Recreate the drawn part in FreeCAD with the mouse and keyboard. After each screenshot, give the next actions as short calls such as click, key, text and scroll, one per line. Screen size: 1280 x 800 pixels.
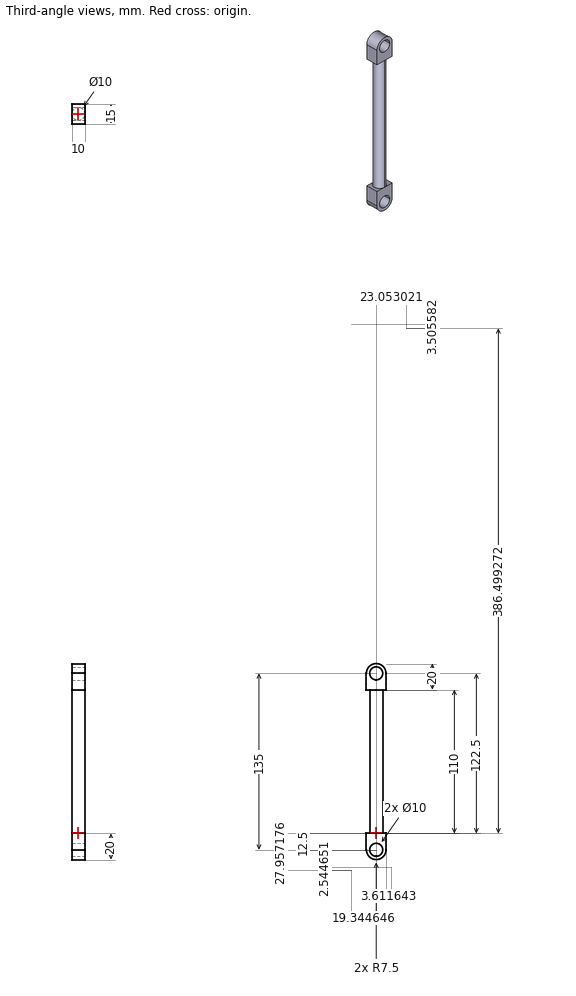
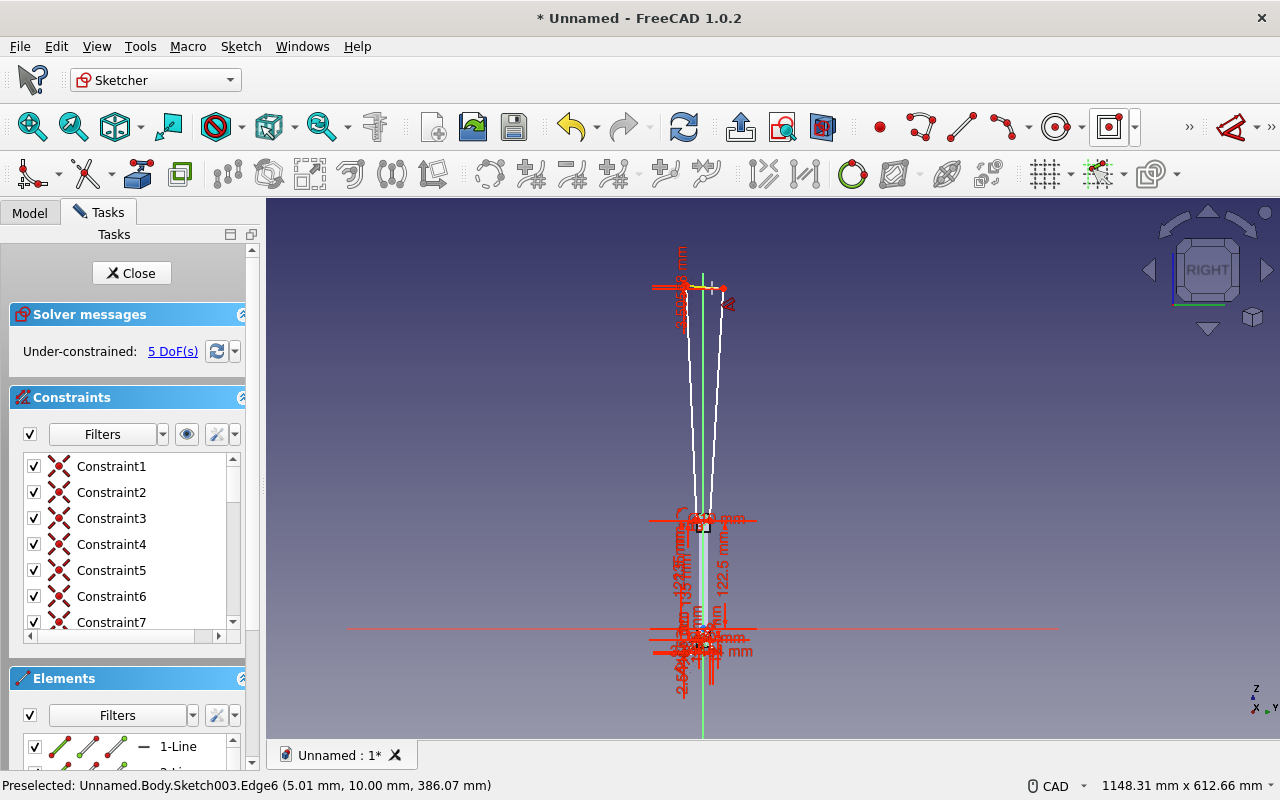
scroll(686, 654, up, 5)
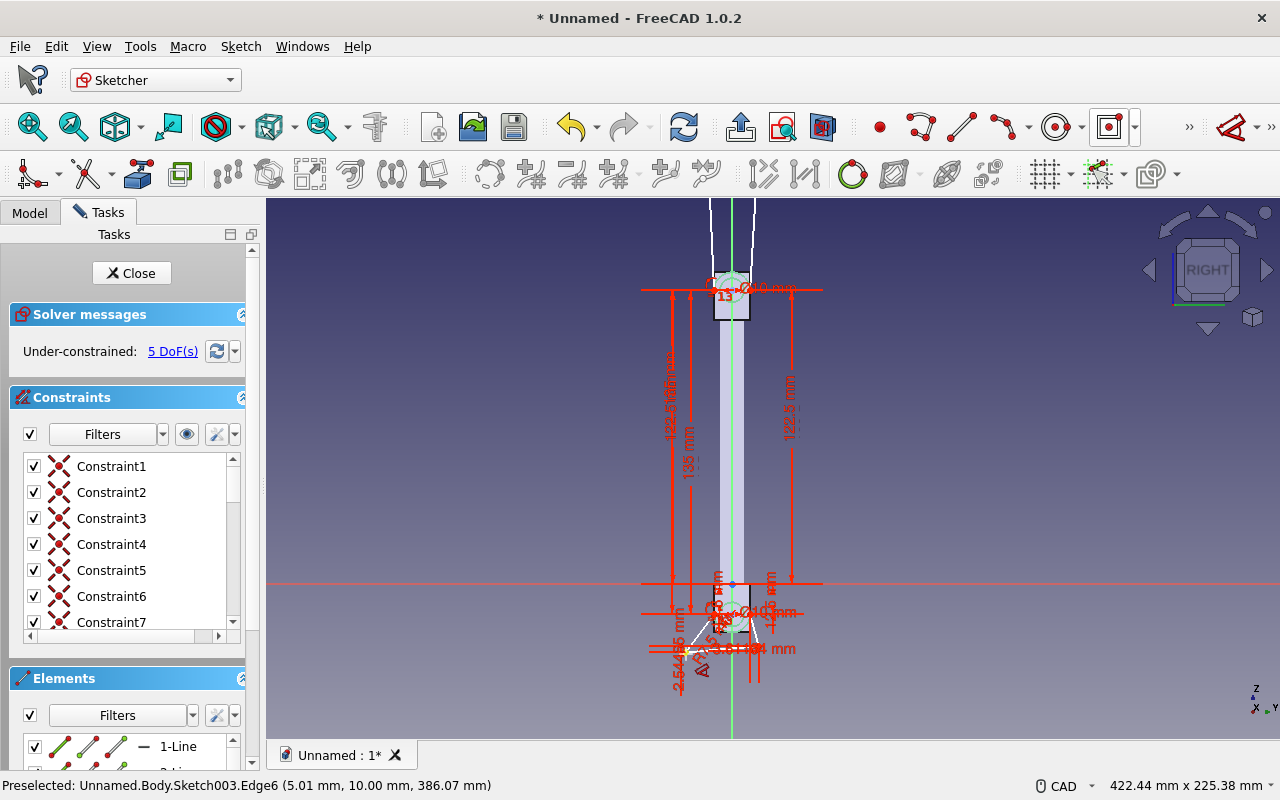
click(686, 652)
click(709, 686)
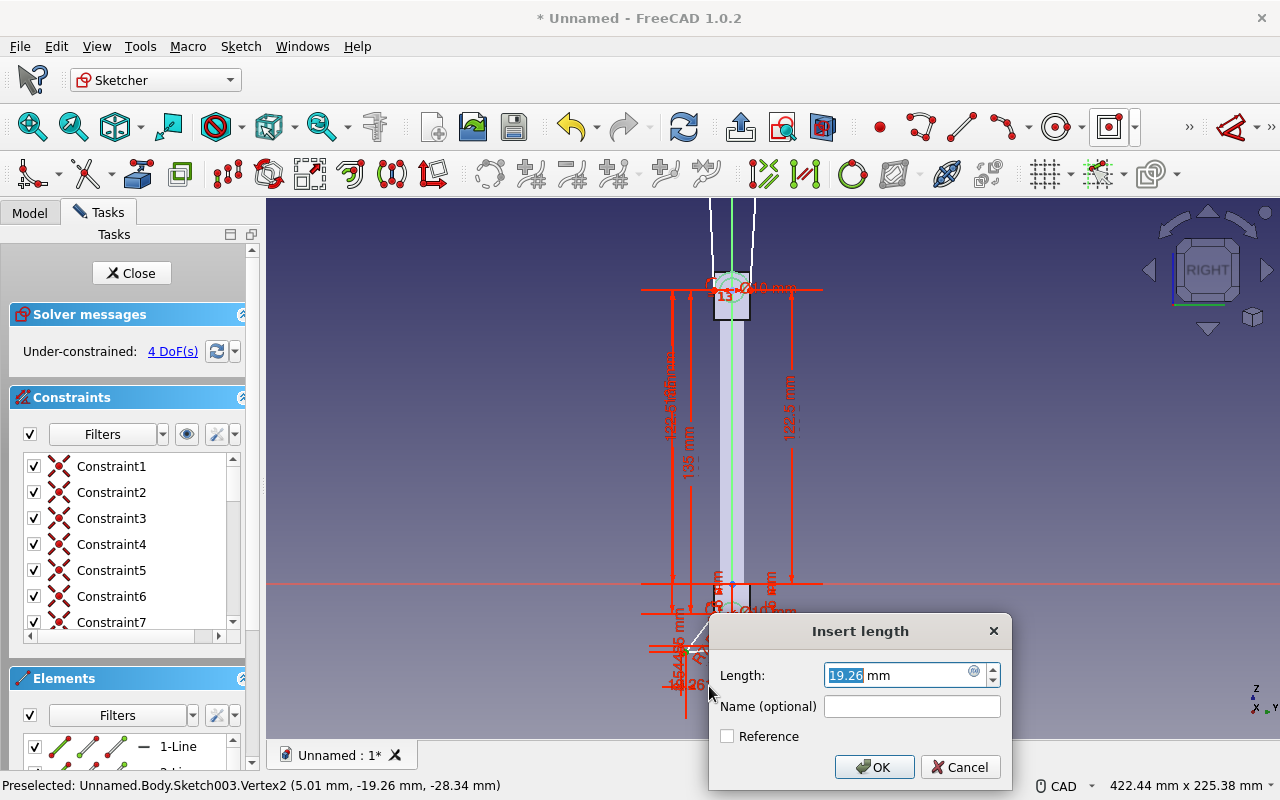
text(19.344646)
key(Return)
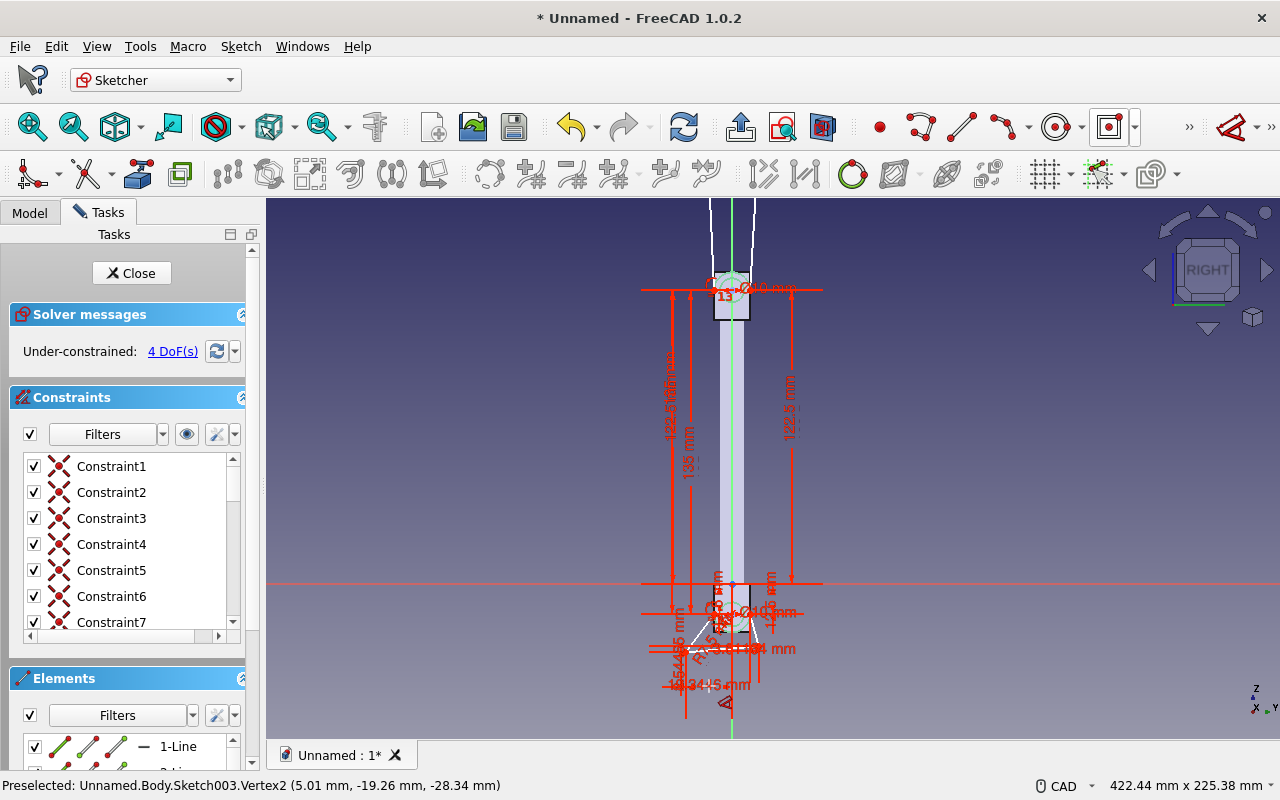
click(686, 652)
click(628, 618)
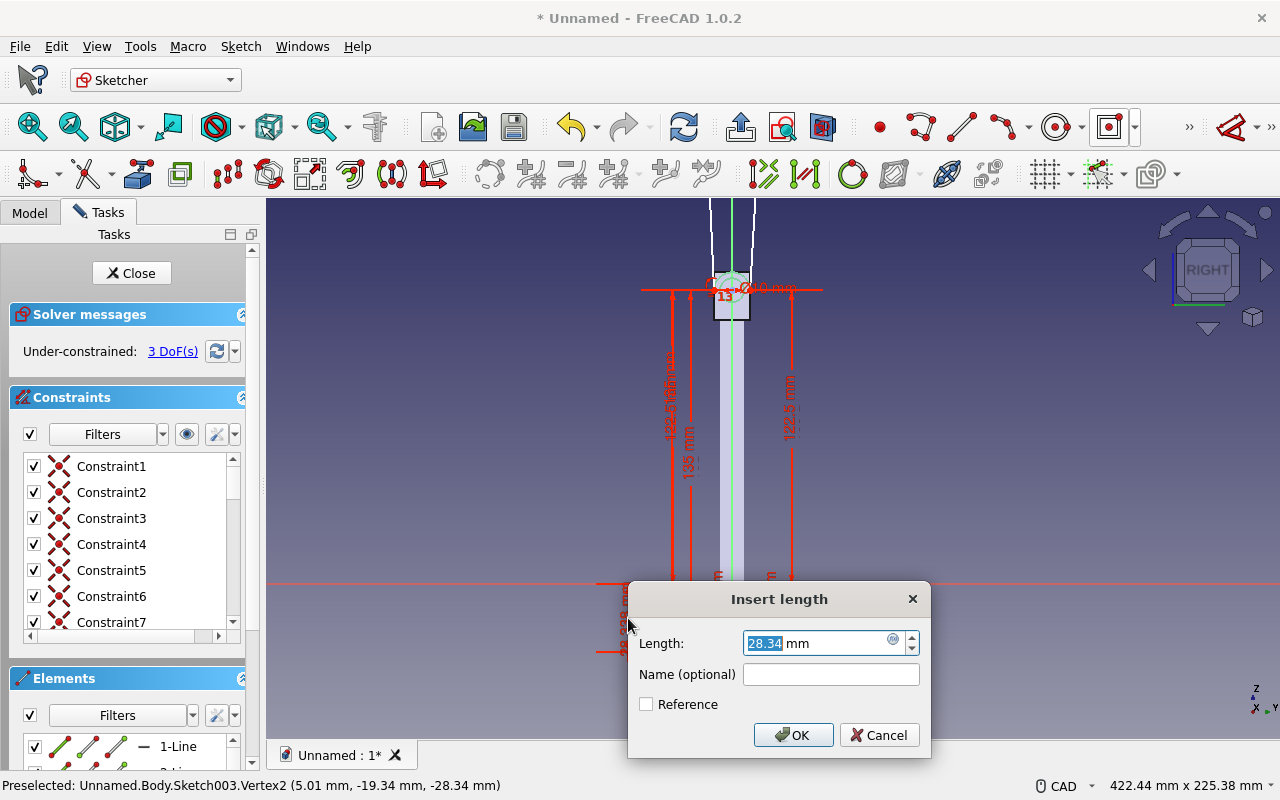
text(27.957176)
key(Return)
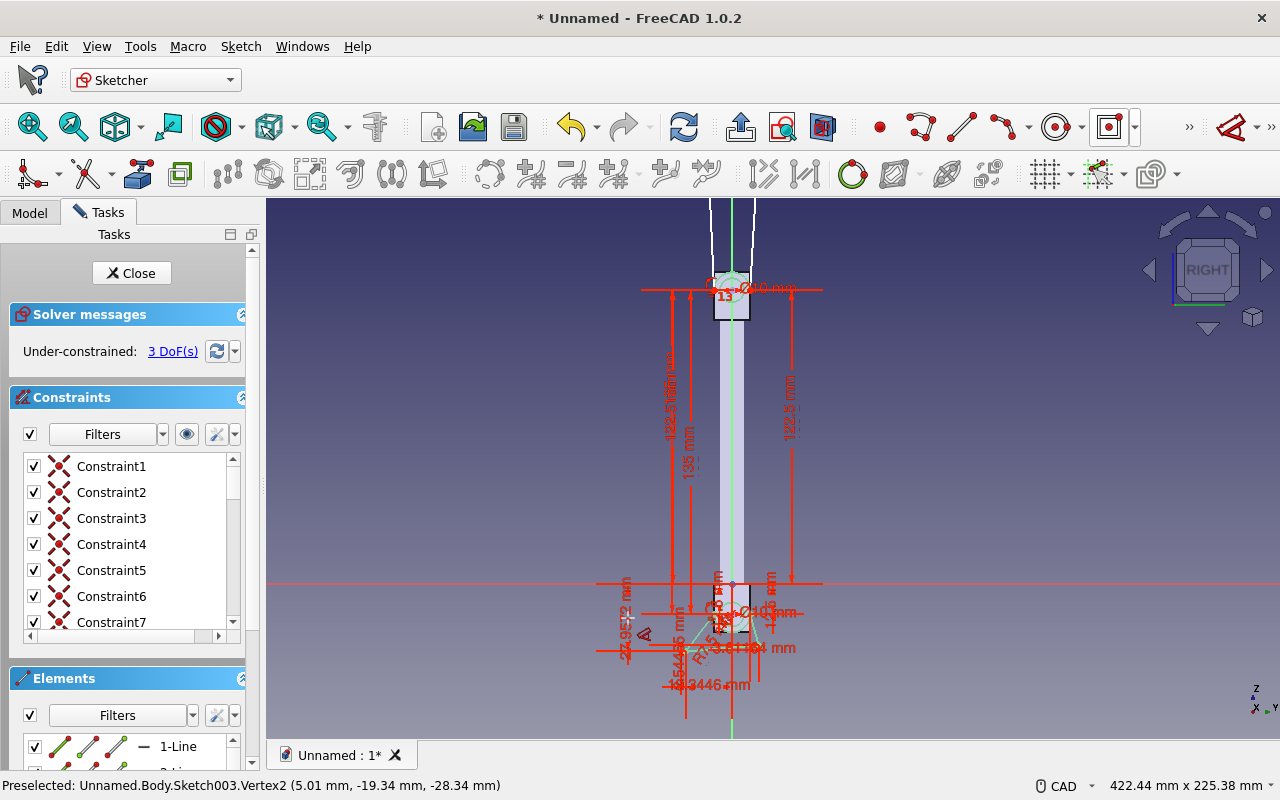
scroll(686, 654, down, 5)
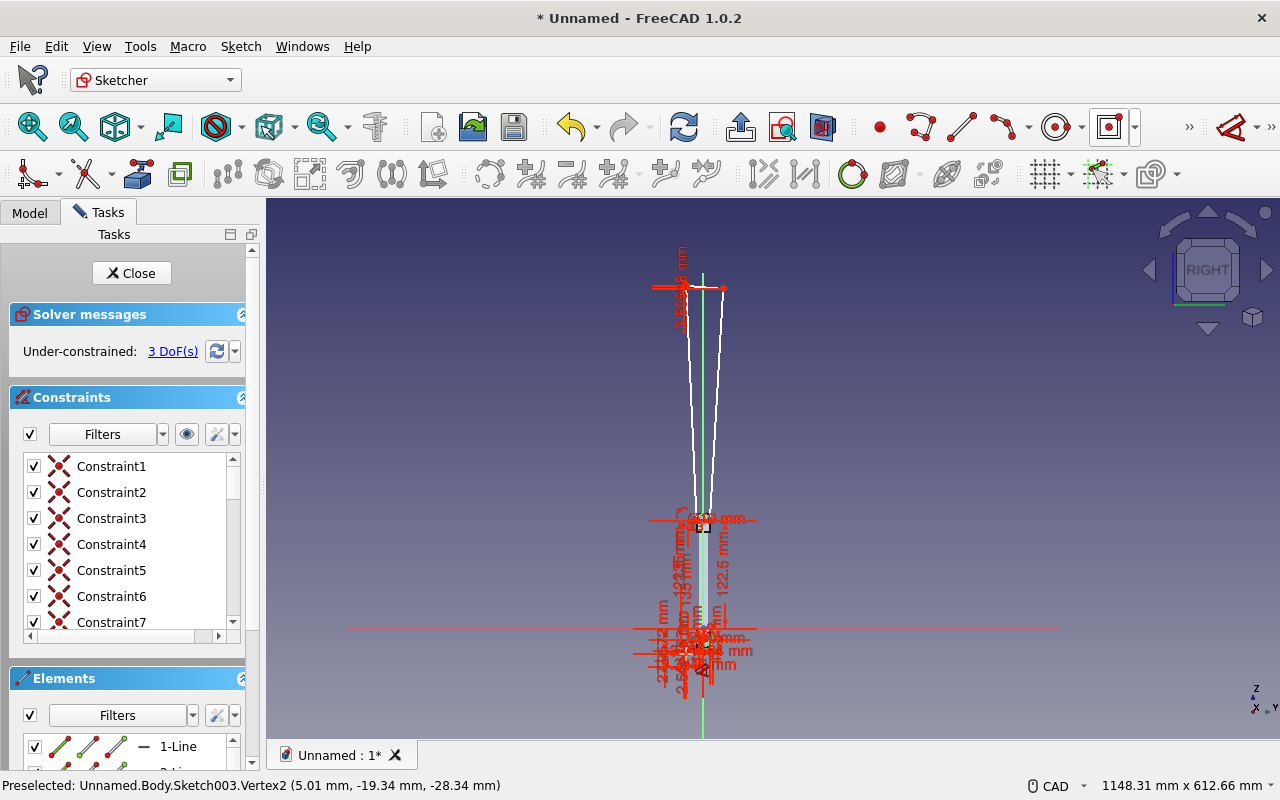
scroll(723, 289, up, 4)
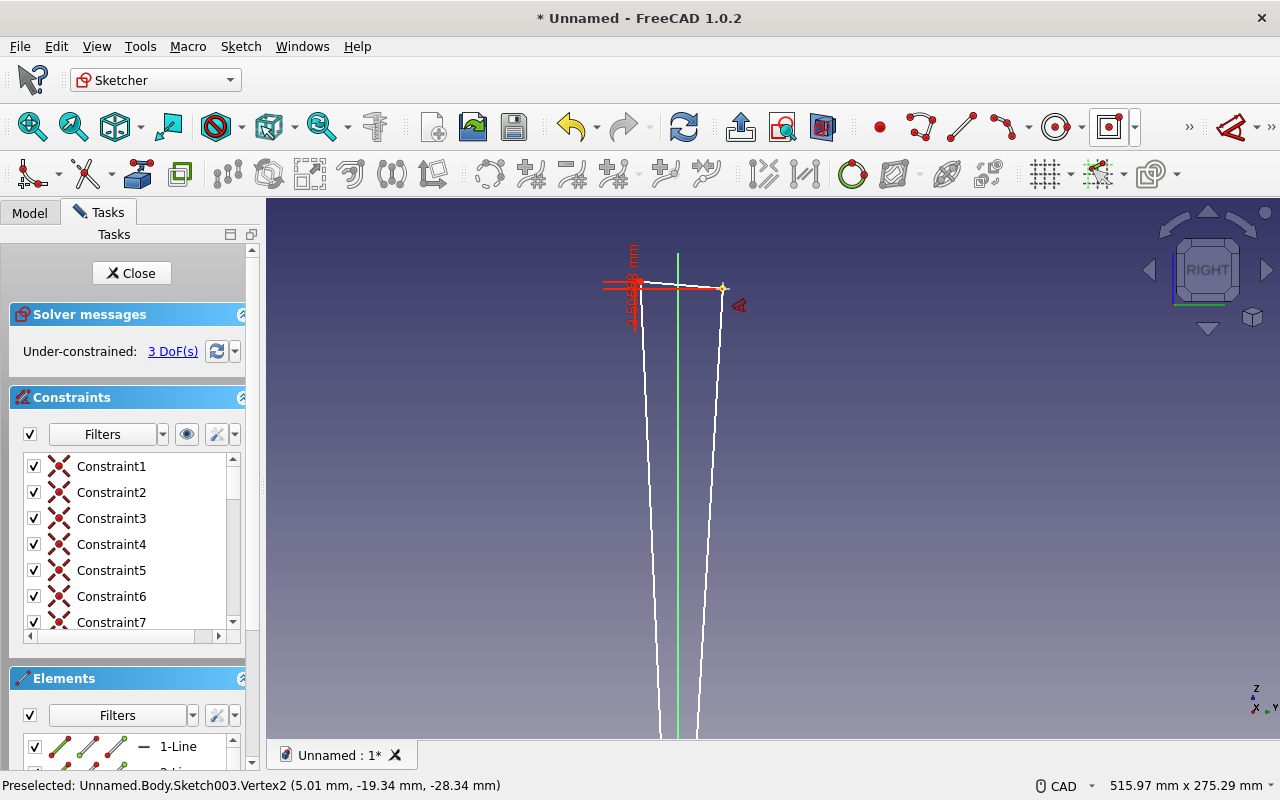
click(723, 289)
click(701, 255)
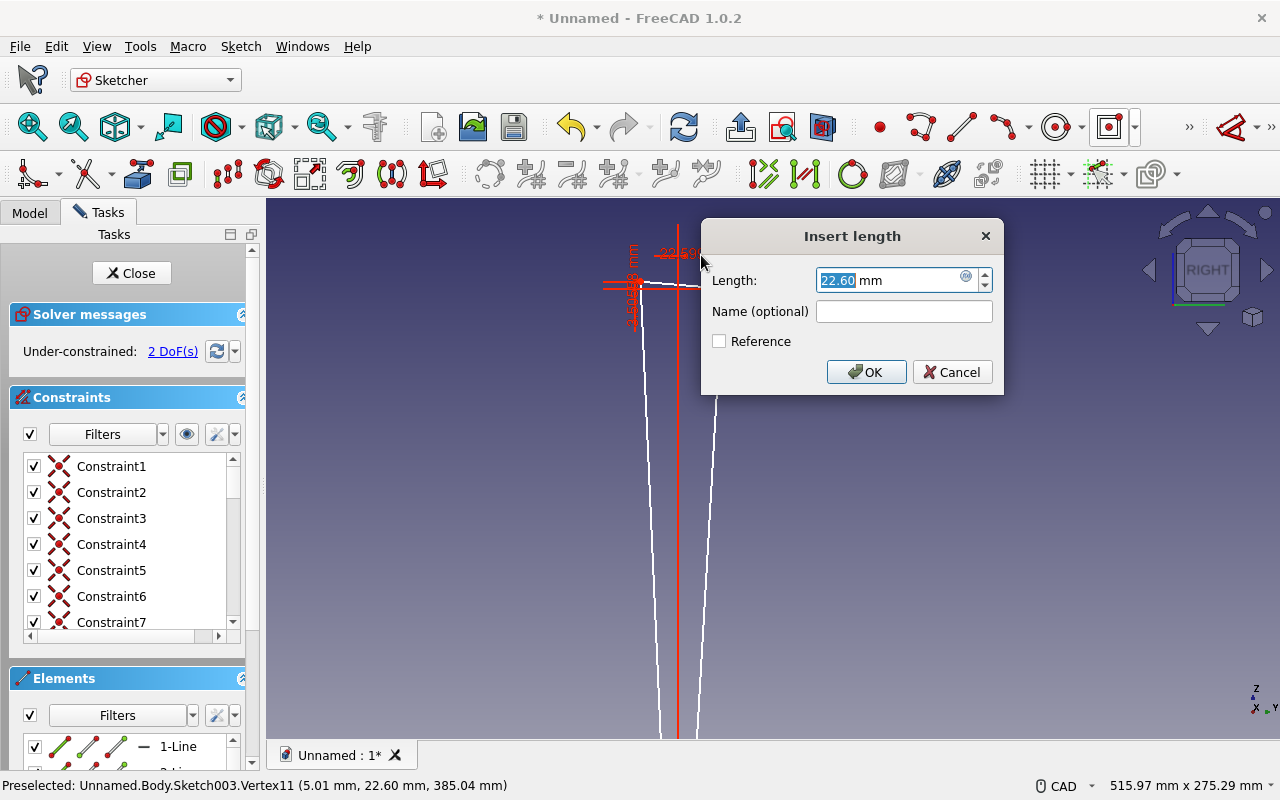
text(23.053021)
key(Return)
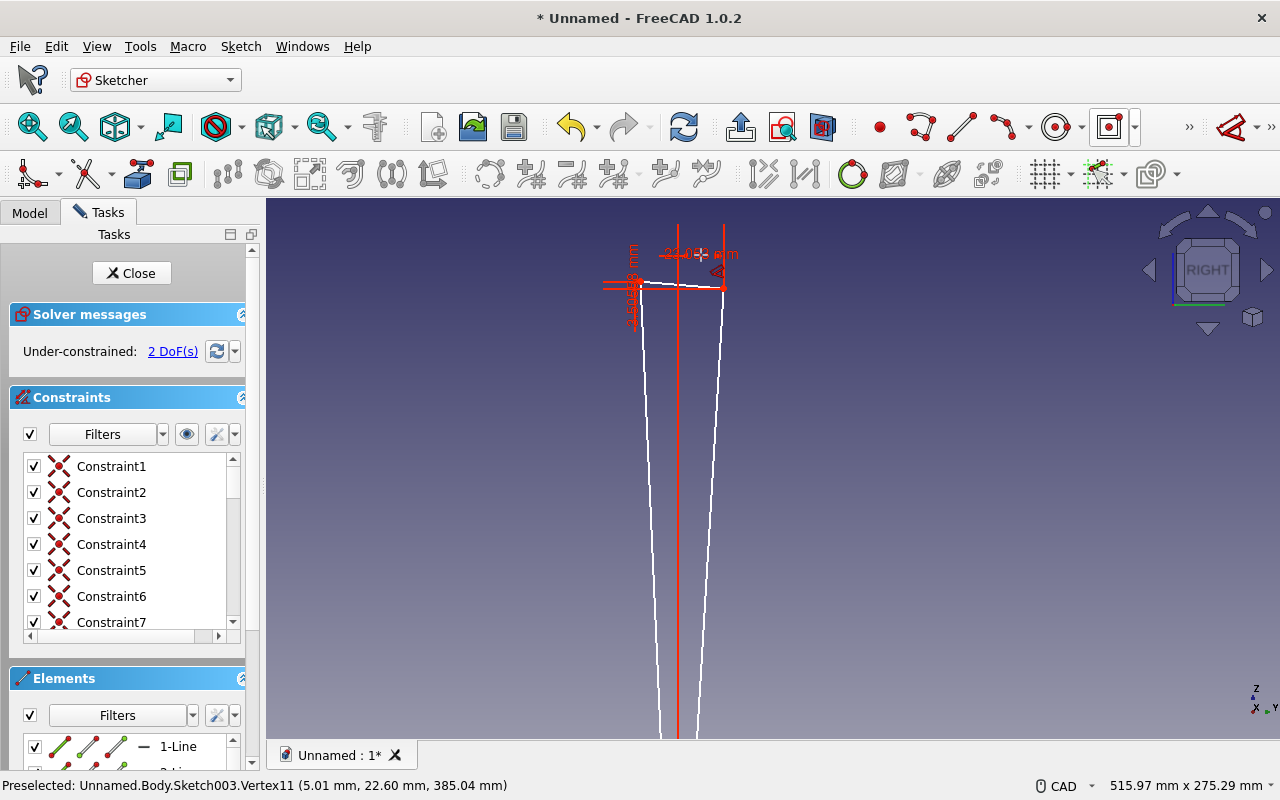
click(640, 282)
click(659, 248)